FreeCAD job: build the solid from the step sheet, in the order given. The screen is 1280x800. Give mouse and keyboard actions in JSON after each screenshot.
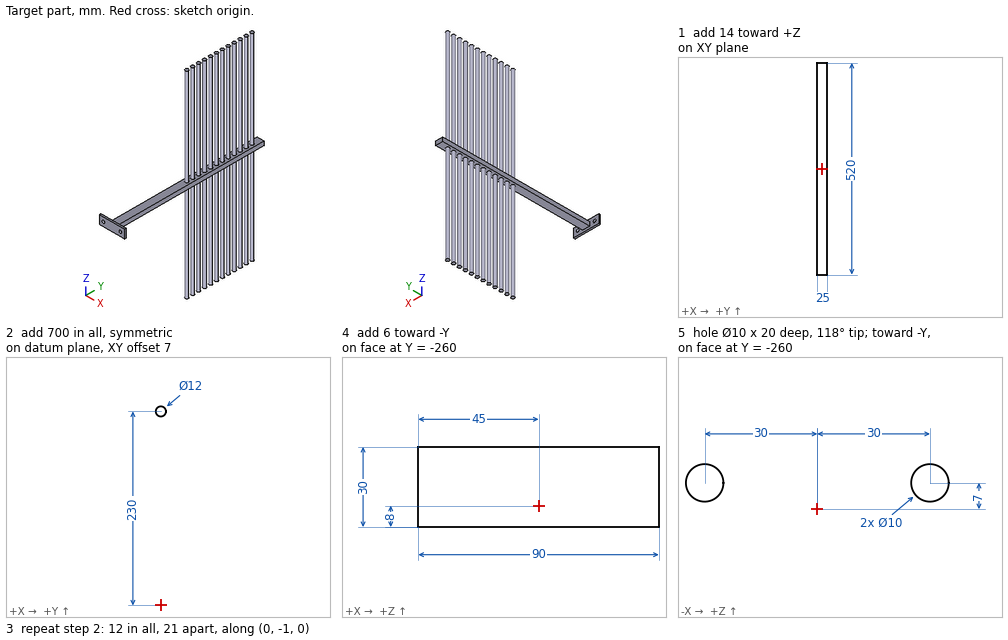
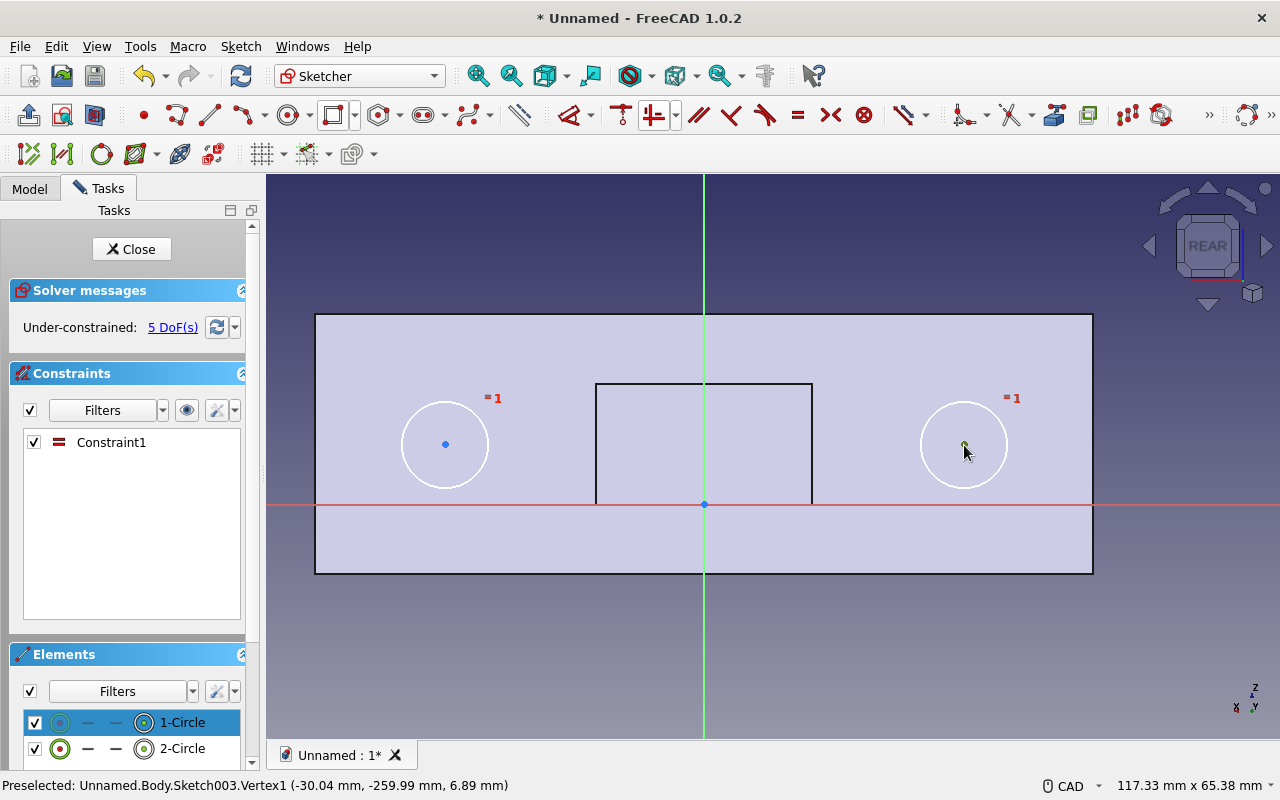
{"action": "left_click", "coordinate": [445, 445]}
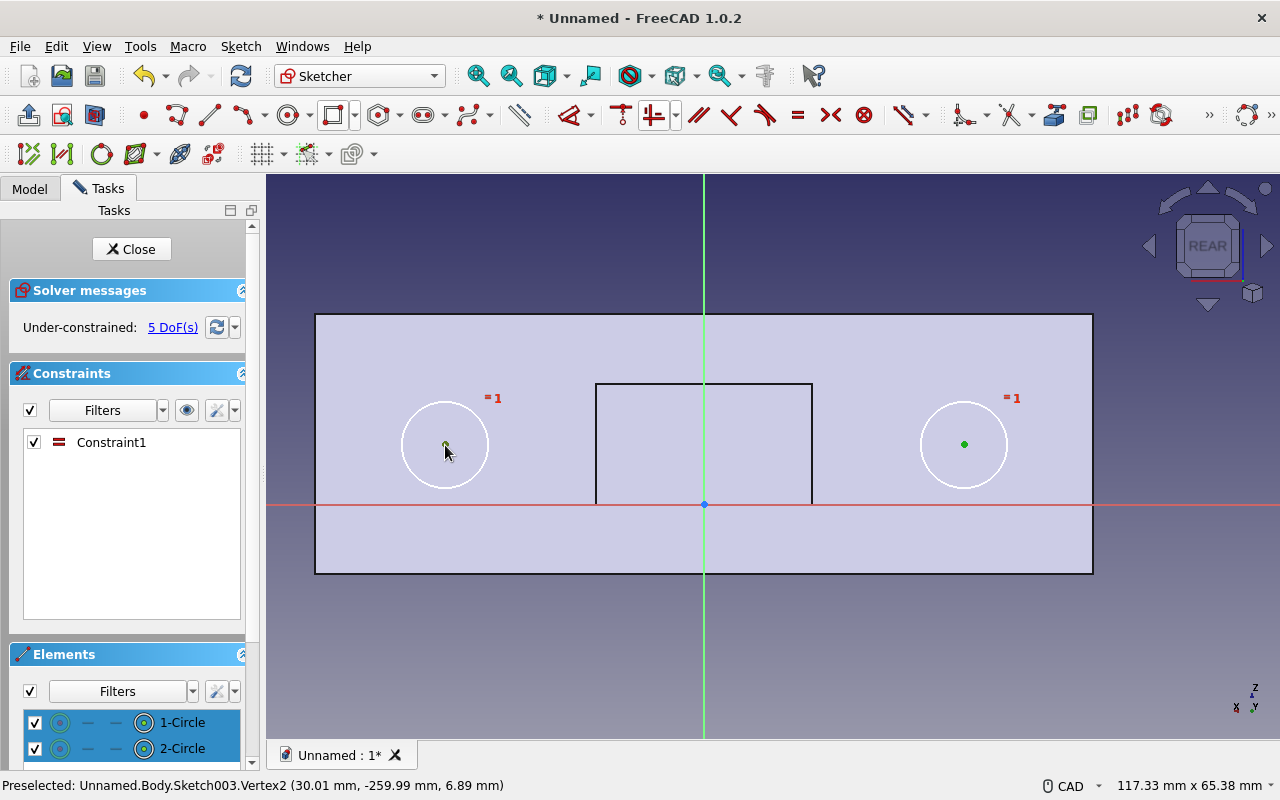
{"action": "left_click", "coordinate": [676, 116]}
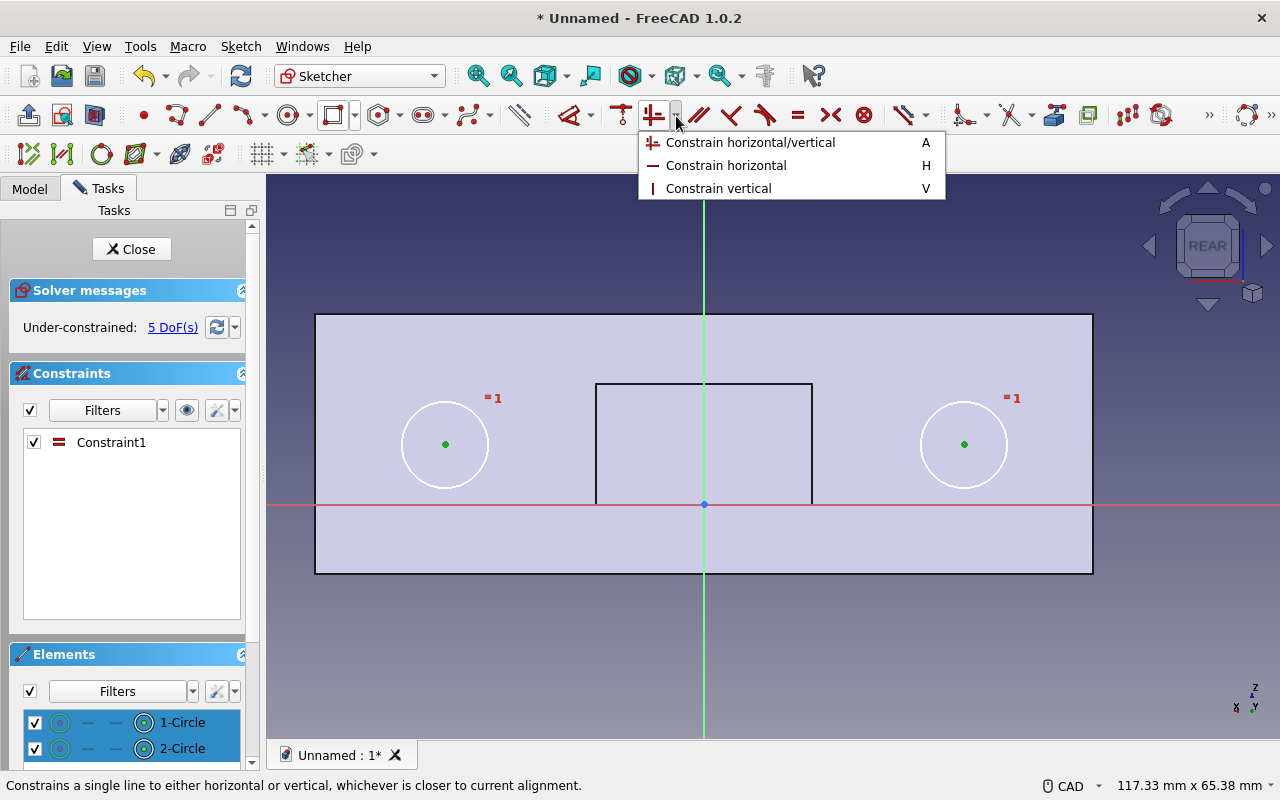
{"action": "left_click", "coordinate": [792, 166]}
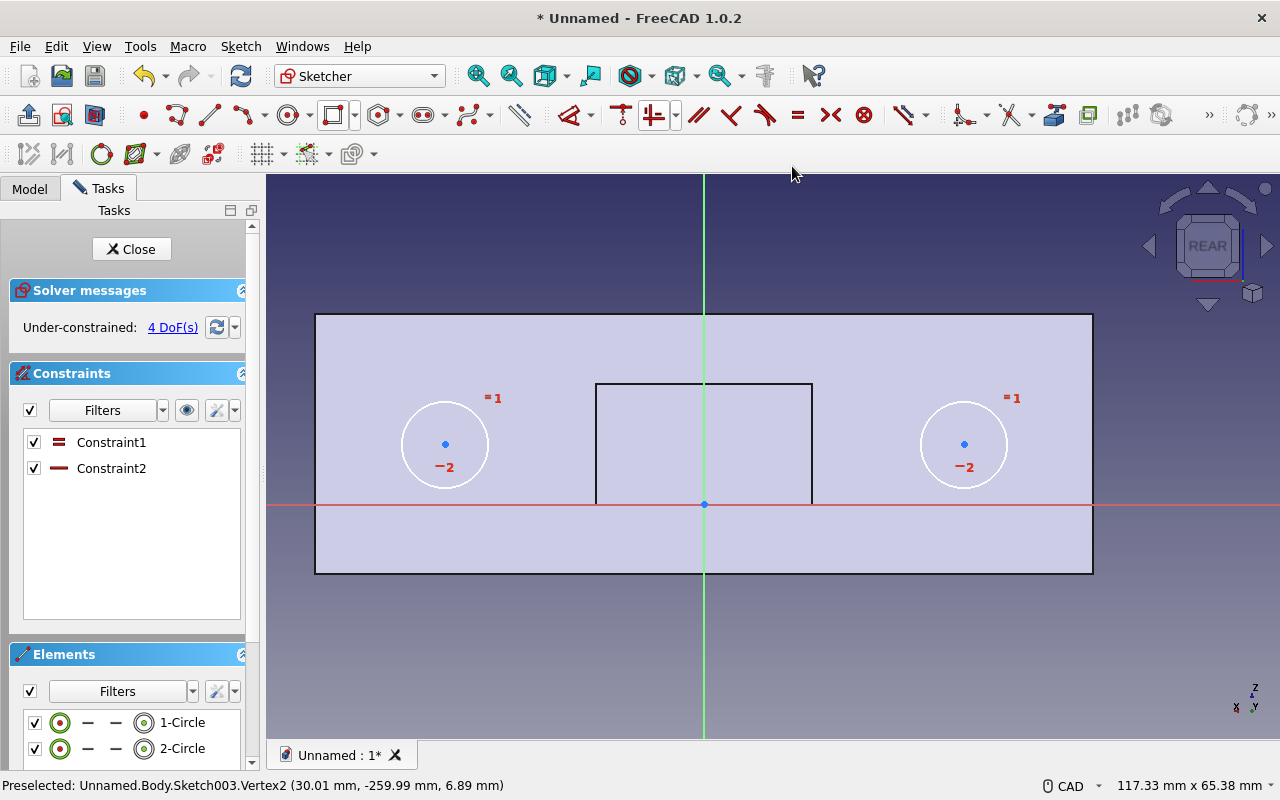
{"action": "left_click", "coordinate": [568, 116]}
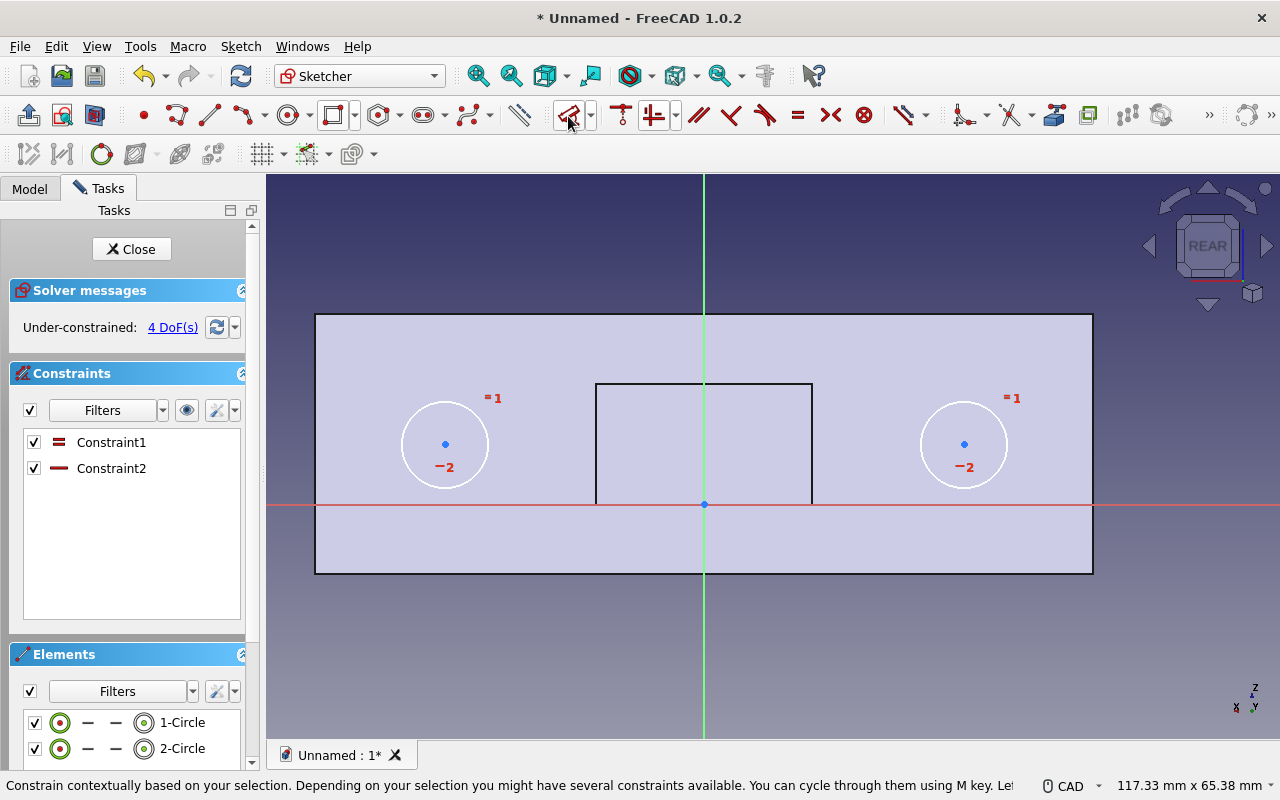
{"action": "left_click", "coordinate": [994, 414]}
{"action": "left_click", "coordinate": [1016, 391]}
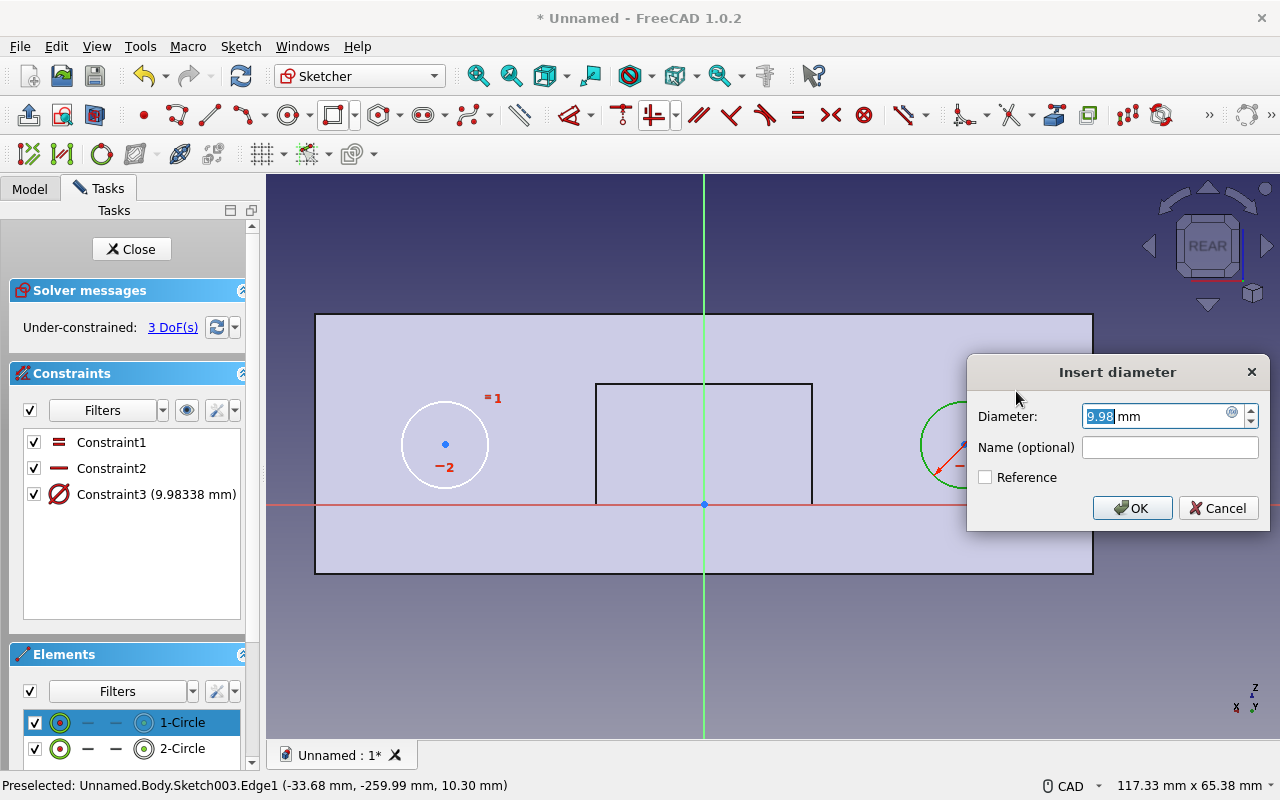
{"action": "type", "text": "10"}
{"action": "key", "text": "Return"}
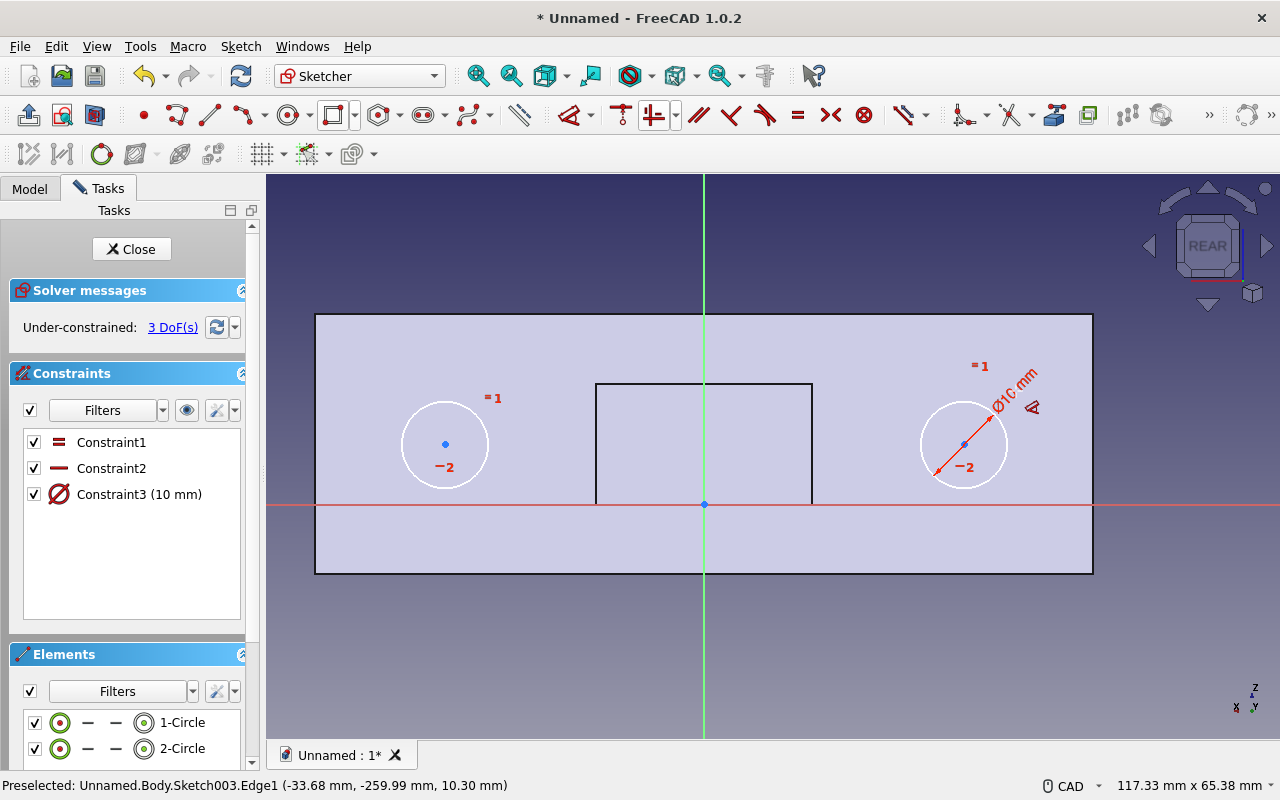
{"action": "left_click", "coordinate": [964, 445]}
{"action": "left_click", "coordinate": [670, 475]}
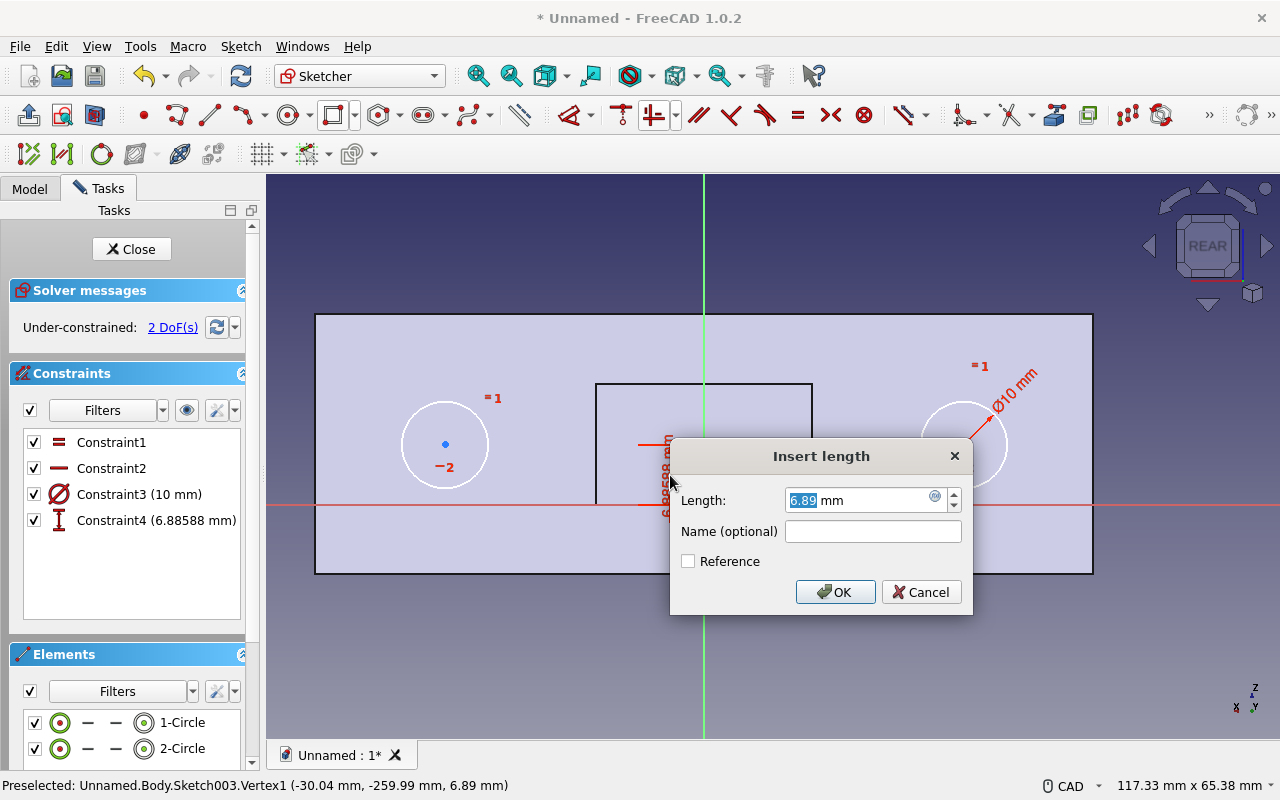
{"action": "type", "text": "7"}
{"action": "key", "text": "Return"}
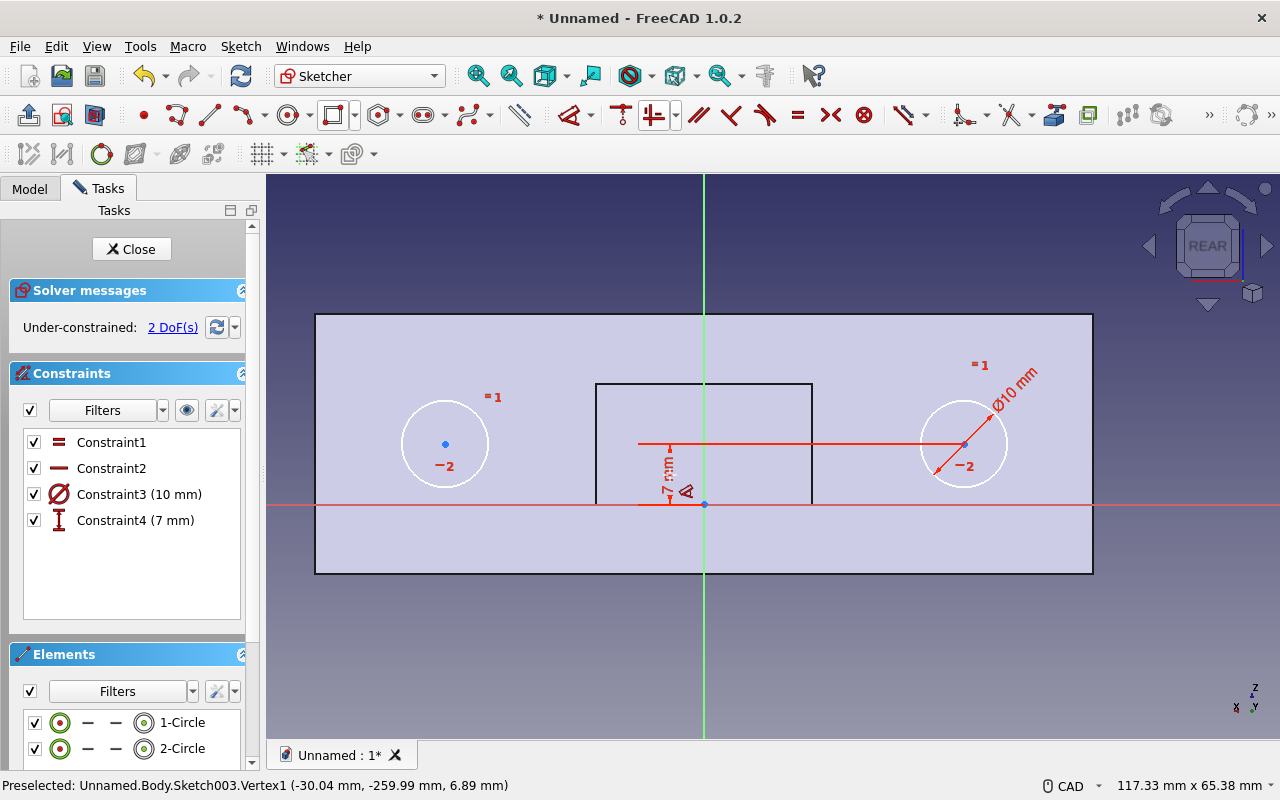
{"action": "left_click", "coordinate": [964, 444]}
{"action": "left_click", "coordinate": [834, 539]}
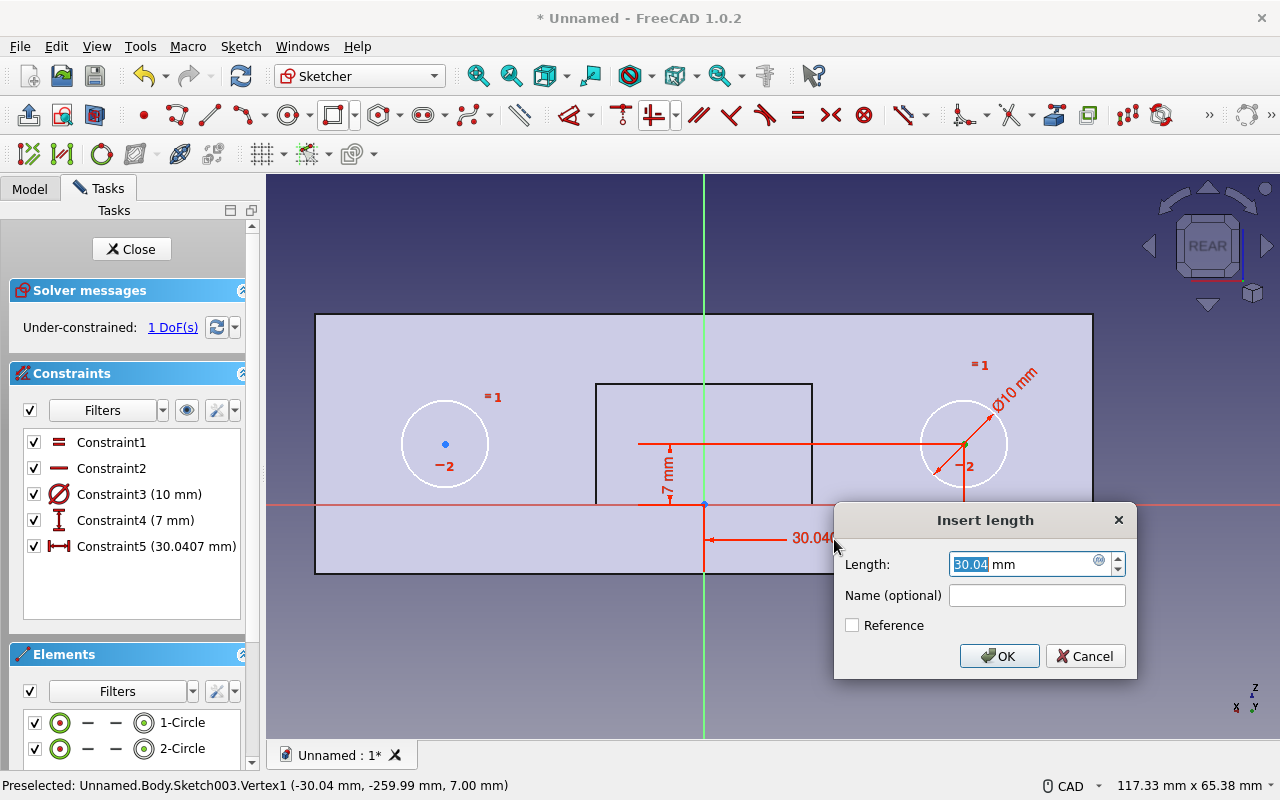
{"action": "type", "text": "30"}
{"action": "key", "text": "Return"}